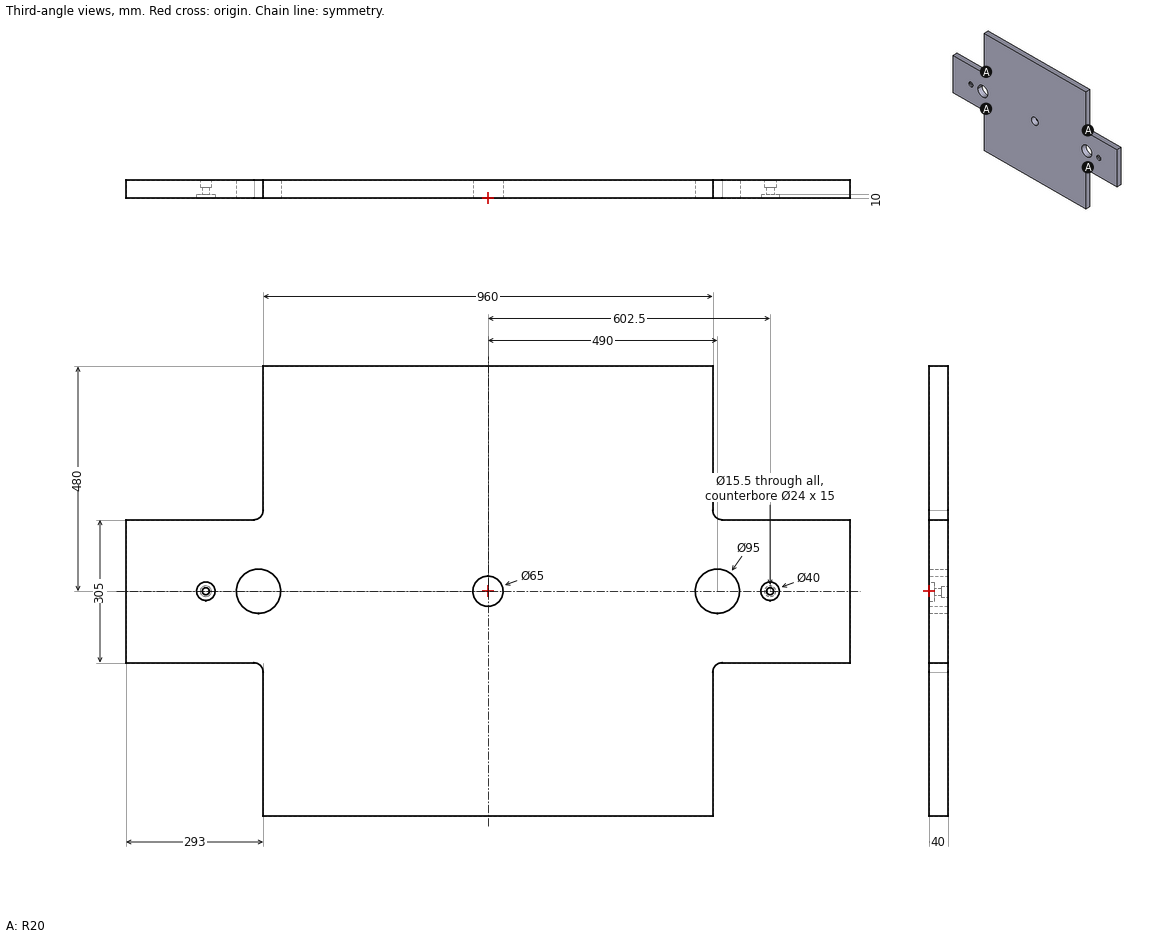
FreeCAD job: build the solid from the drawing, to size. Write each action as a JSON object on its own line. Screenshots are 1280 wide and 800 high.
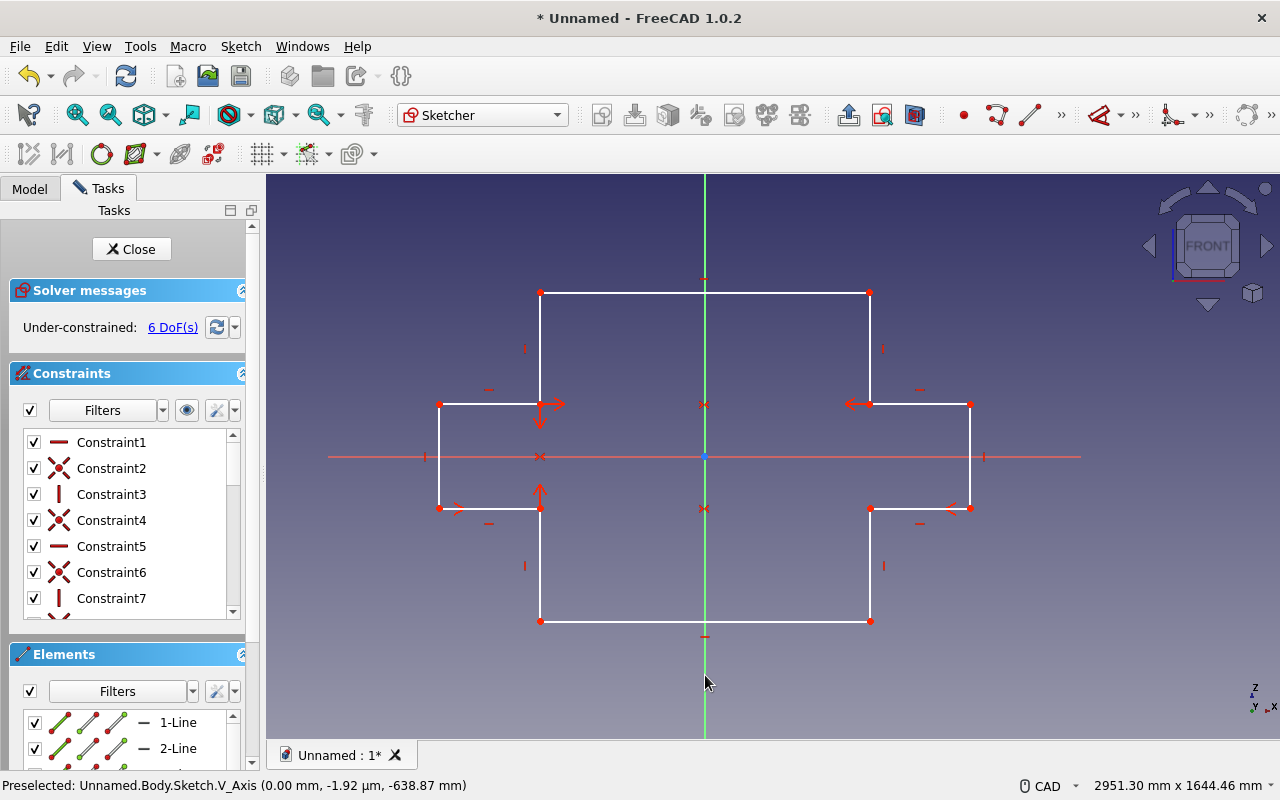
{"action": "left_click", "coordinate": [870, 293]}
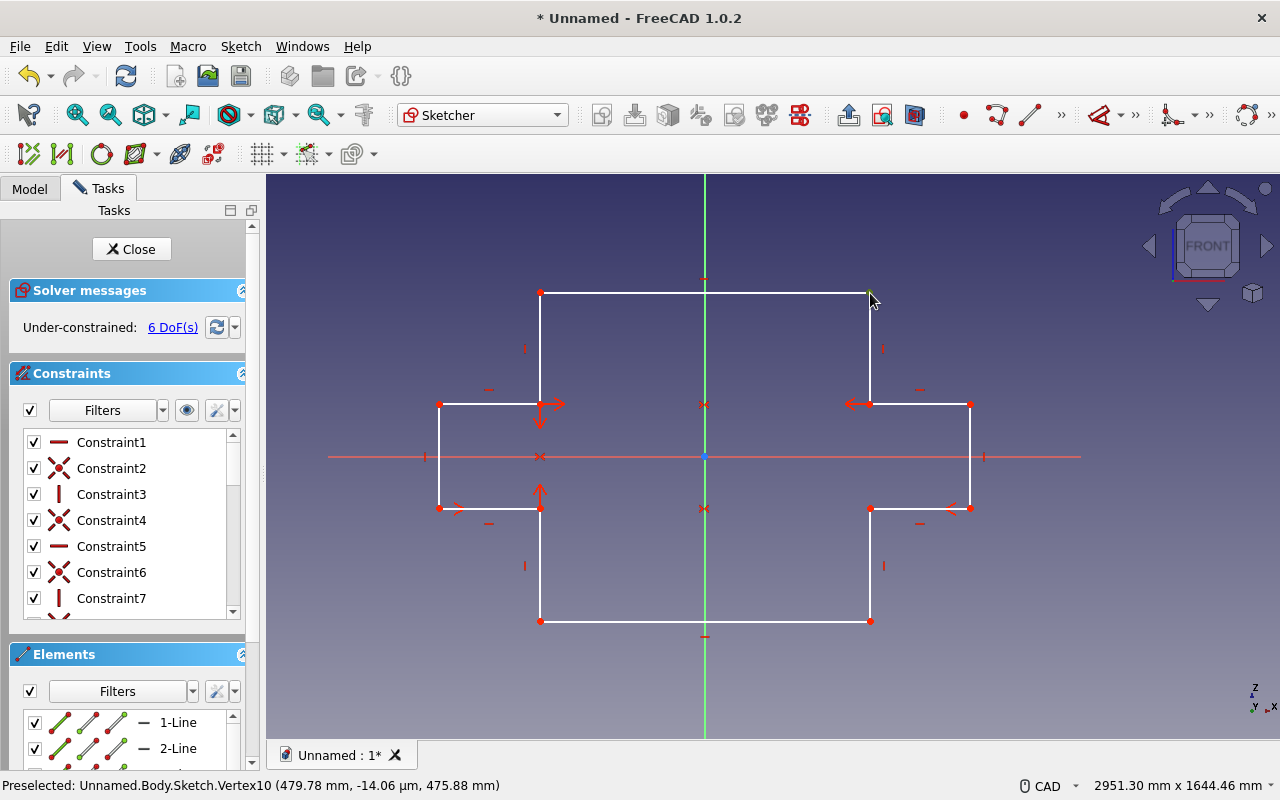
{"action": "left_click", "coordinate": [870, 622]}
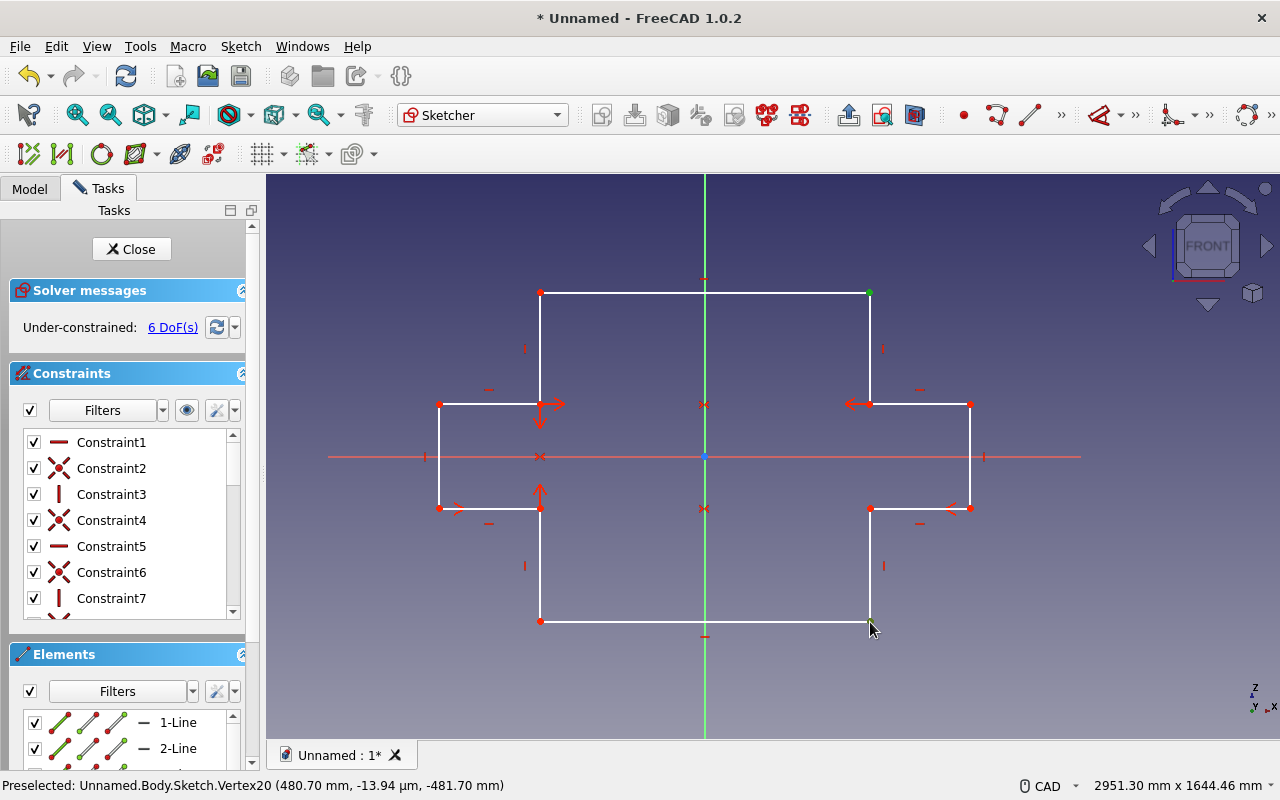
{"action": "left_click", "coordinate": [353, 456]}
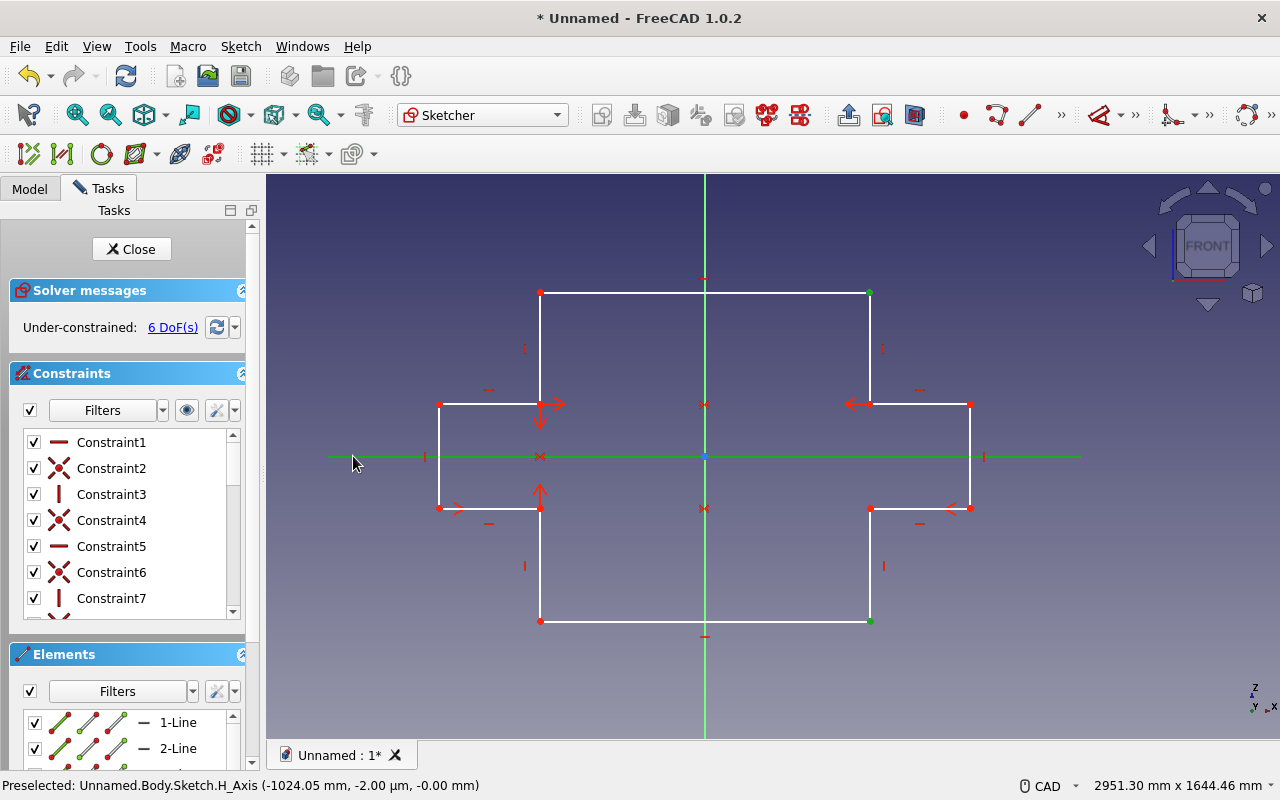
{"action": "key", "text": "s"}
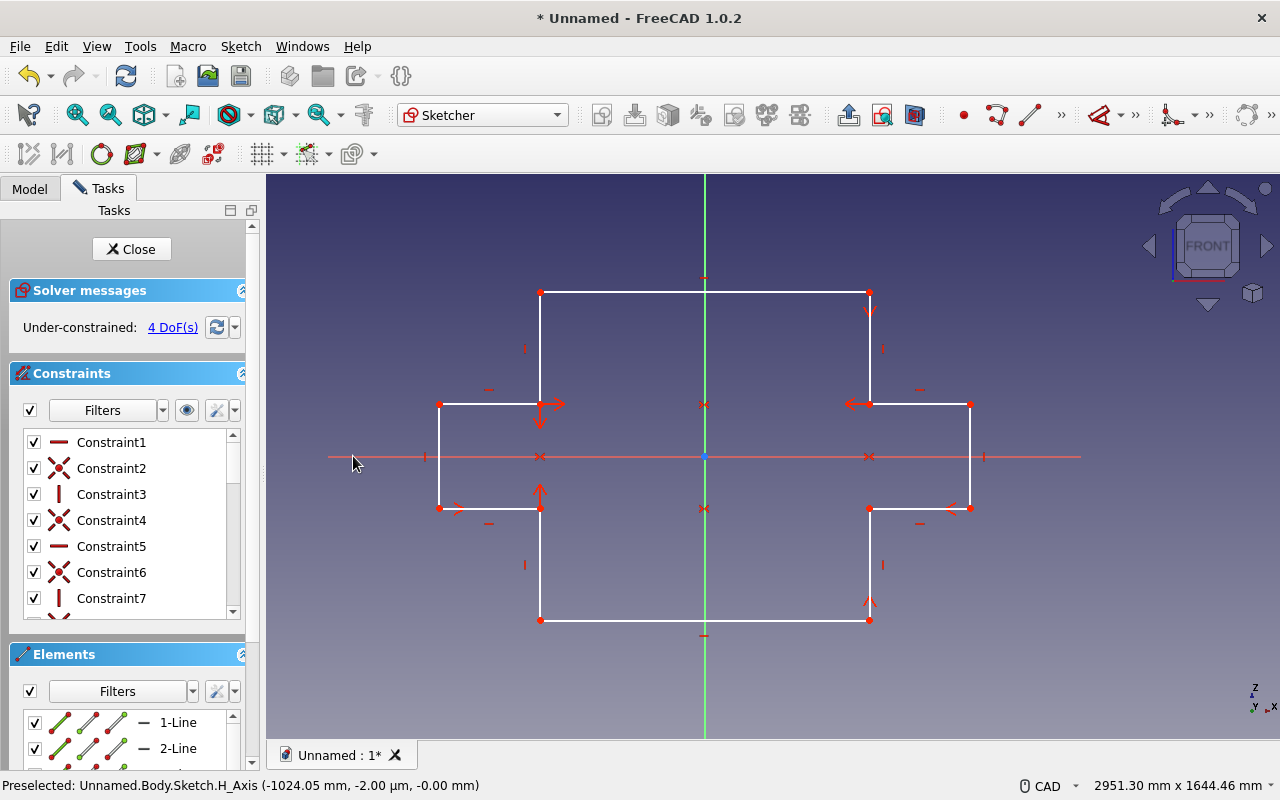
{"action": "left_click", "coordinate": [510, 509]}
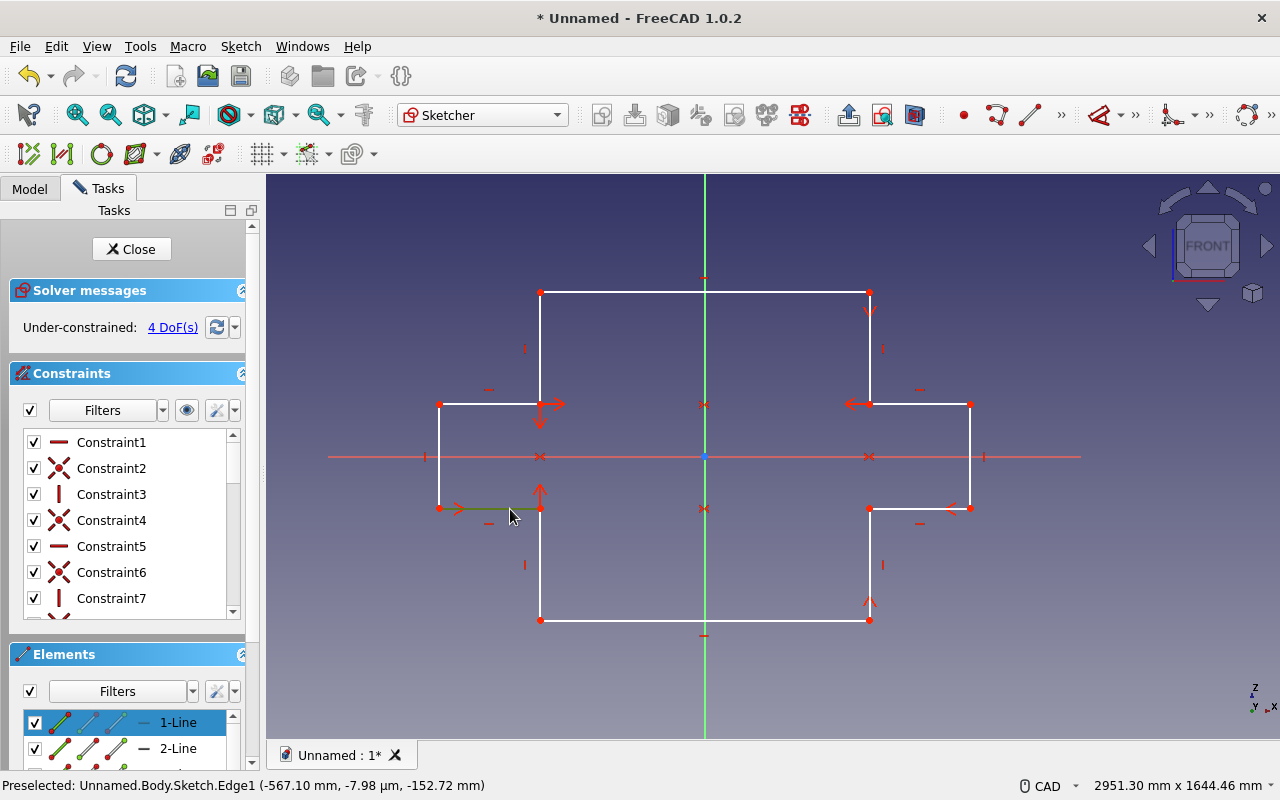
{"action": "left_click", "coordinate": [1120, 116]}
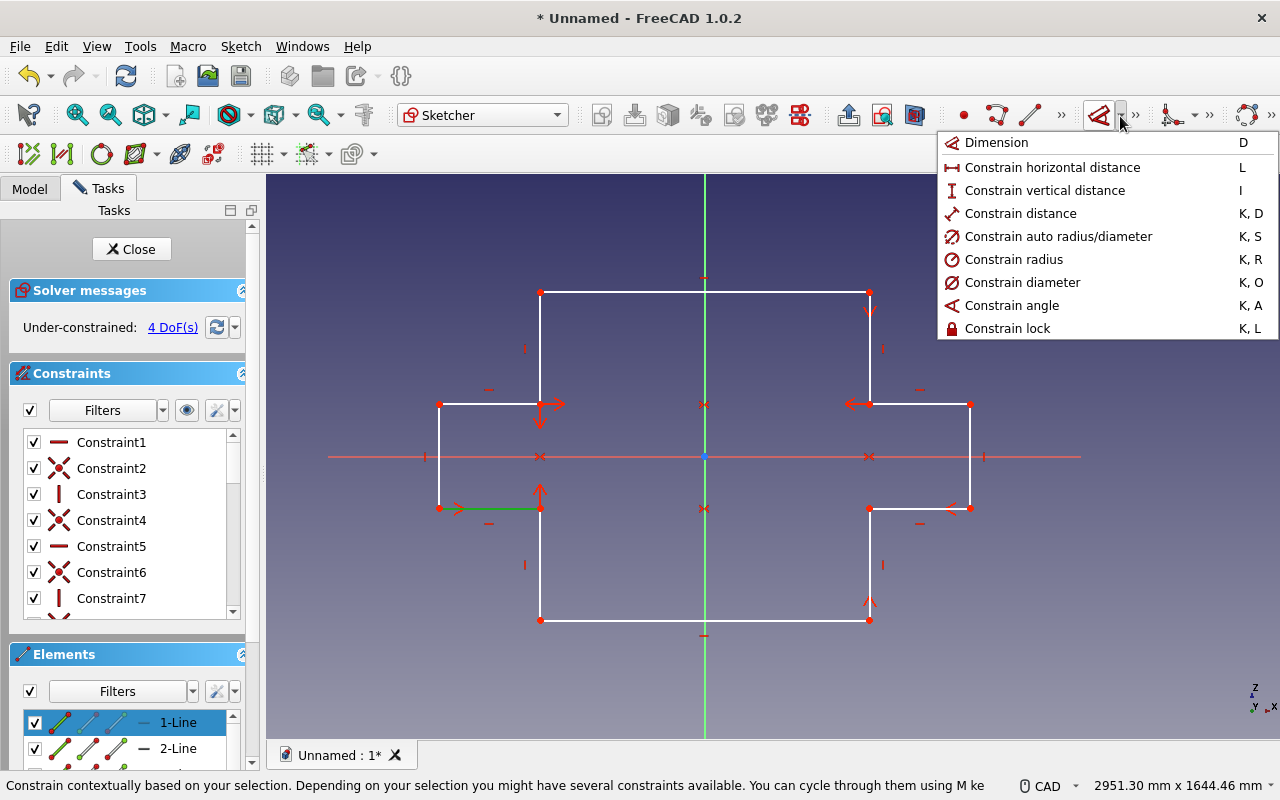
{"action": "left_click", "coordinate": [1108, 168]}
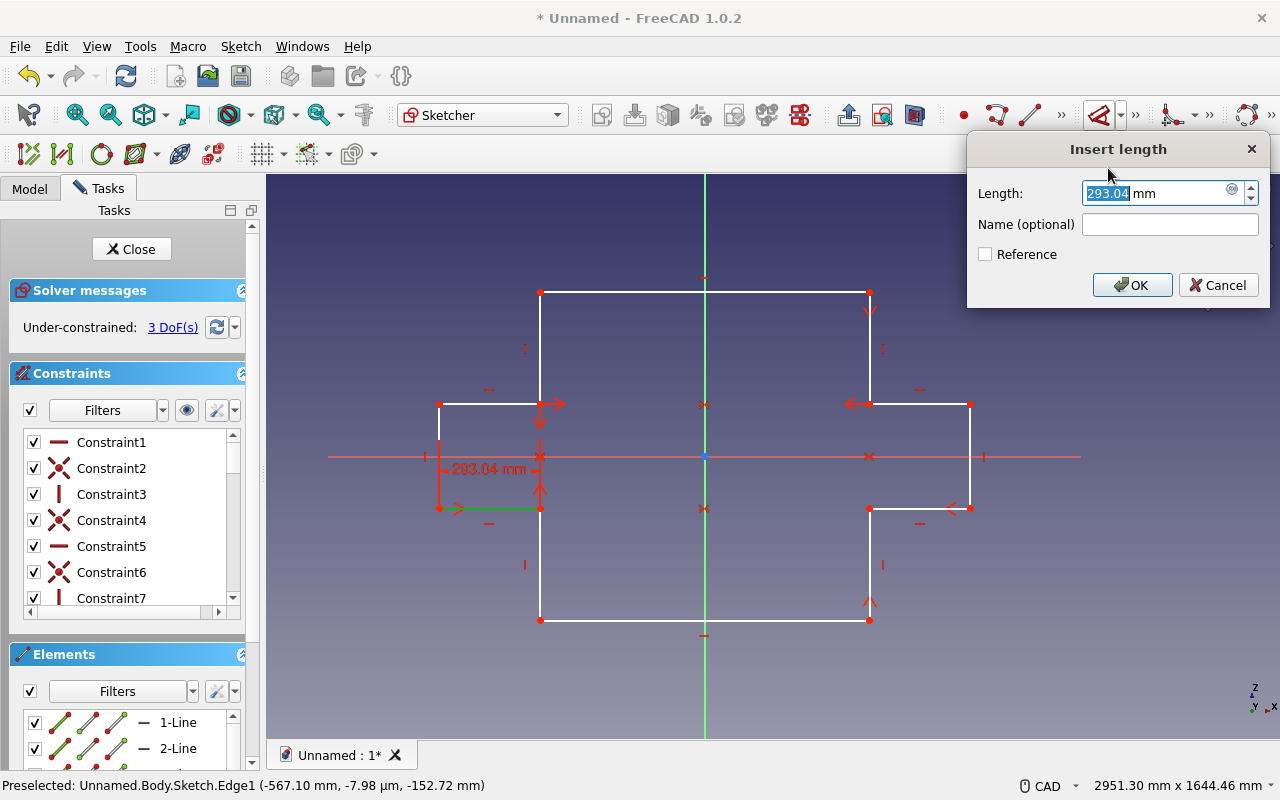
{"action": "type", "text": "293"}
{"action": "key", "text": "Return"}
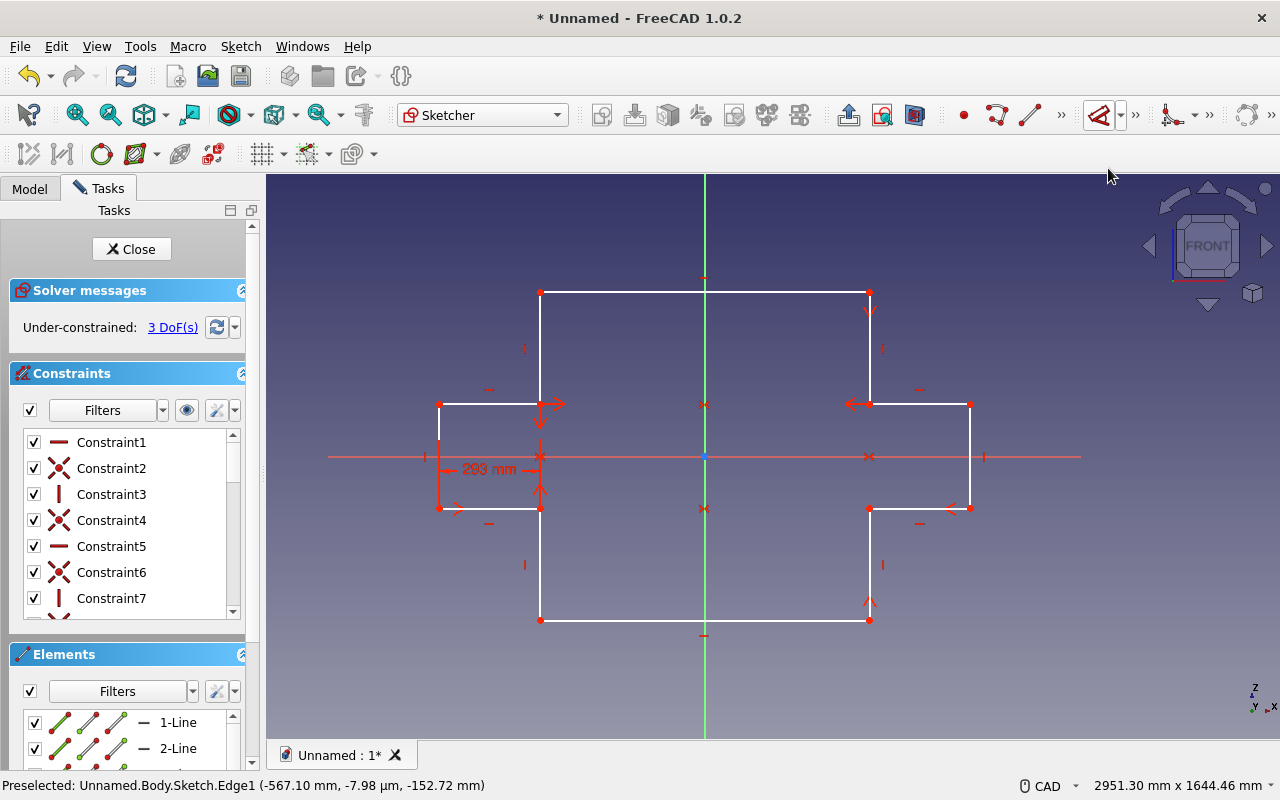
{"action": "left_click", "coordinate": [439, 477]}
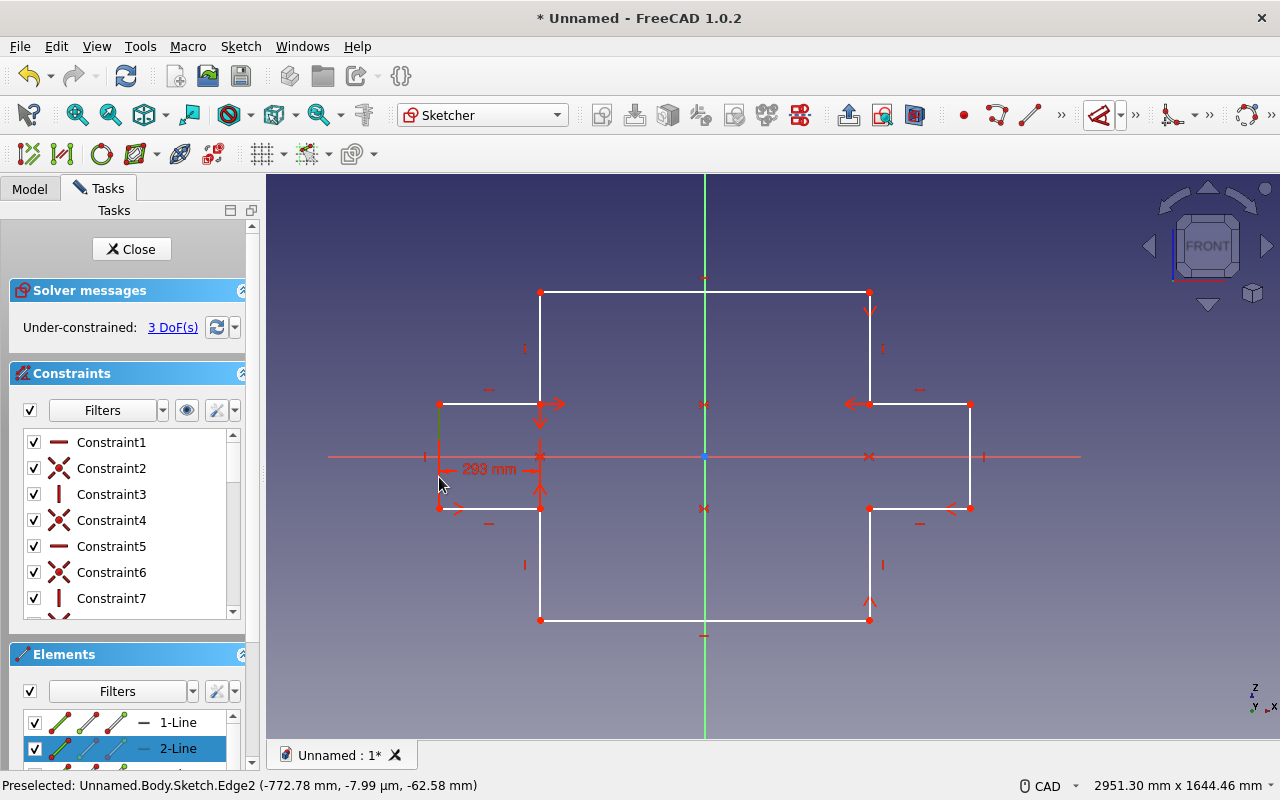
{"action": "left_click", "coordinate": [1120, 116]}